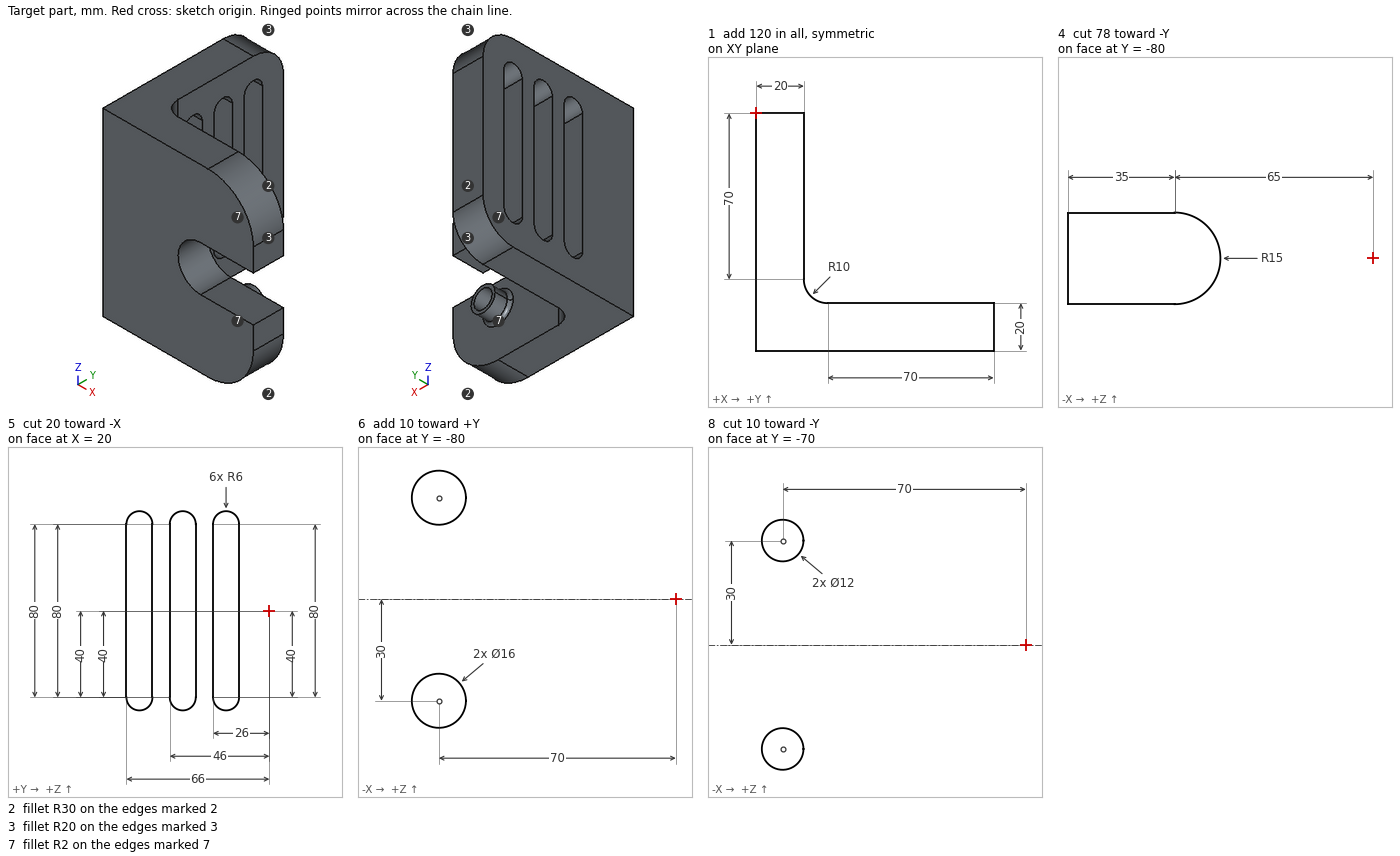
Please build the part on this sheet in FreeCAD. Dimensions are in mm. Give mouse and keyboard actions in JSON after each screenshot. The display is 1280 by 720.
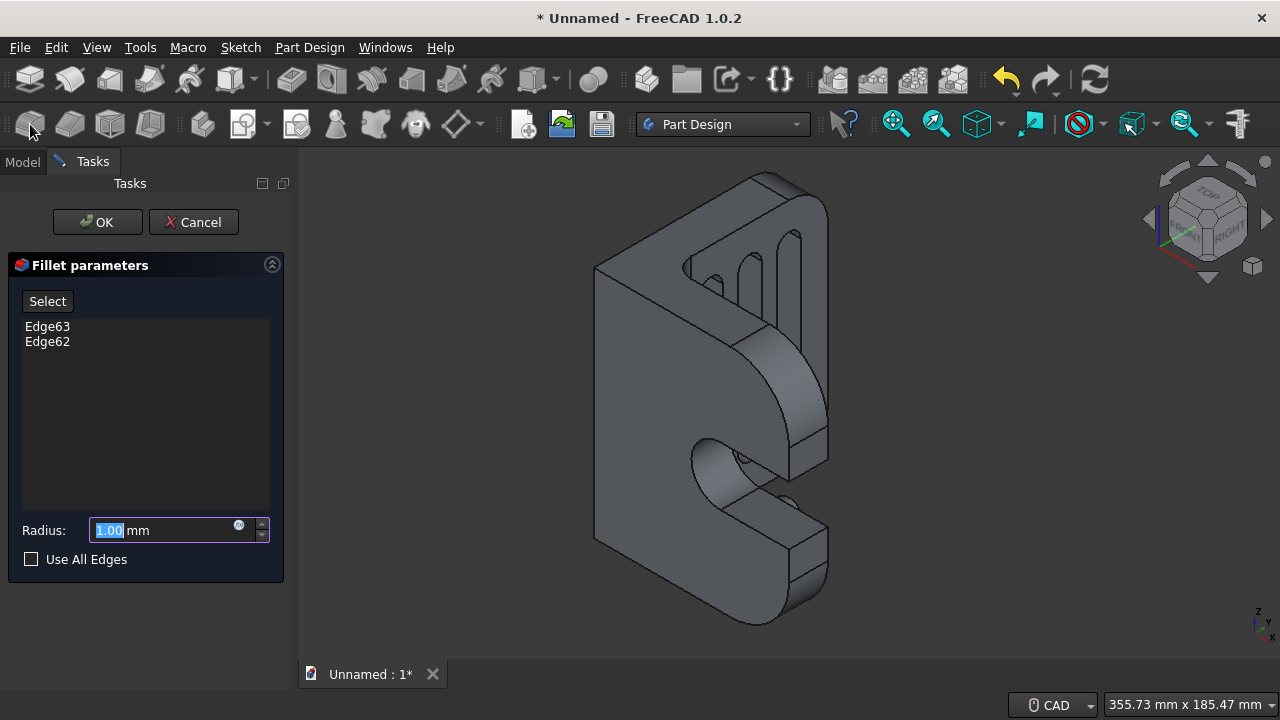
{"action": "type", "text": "2"}
{"action": "key", "text": "Tab"}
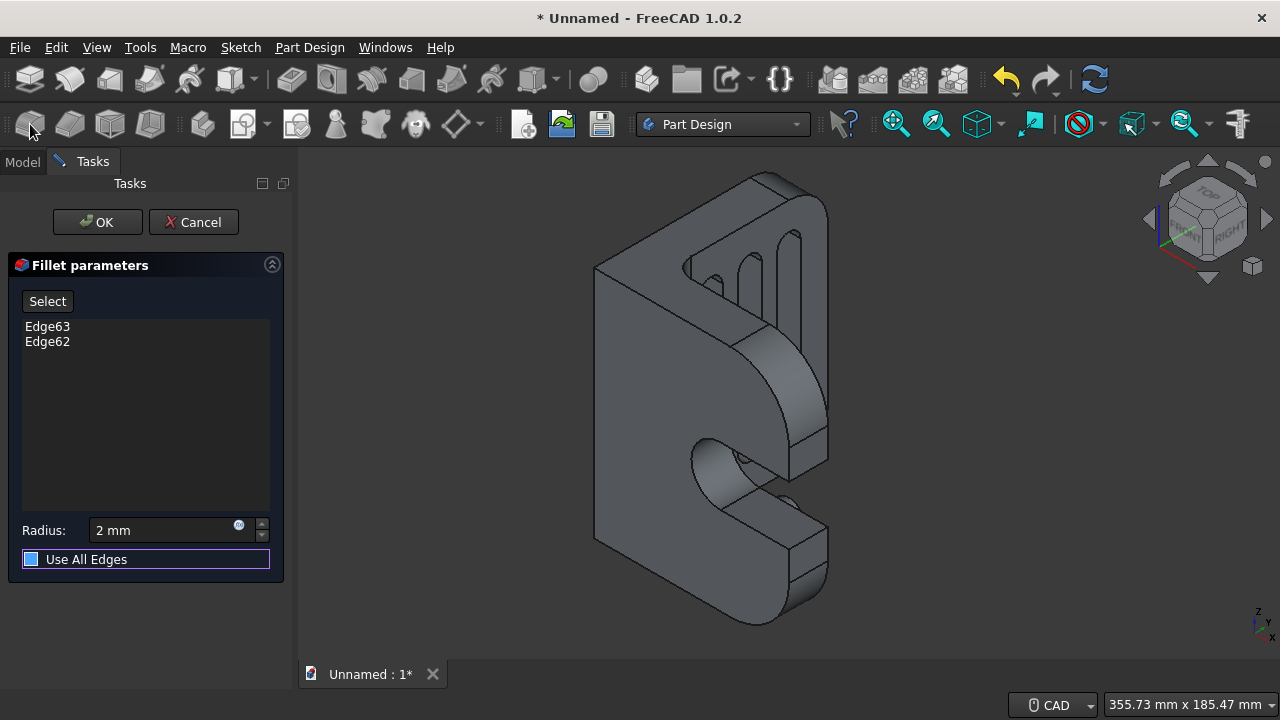
{"action": "left_click", "coordinate": [98, 222]}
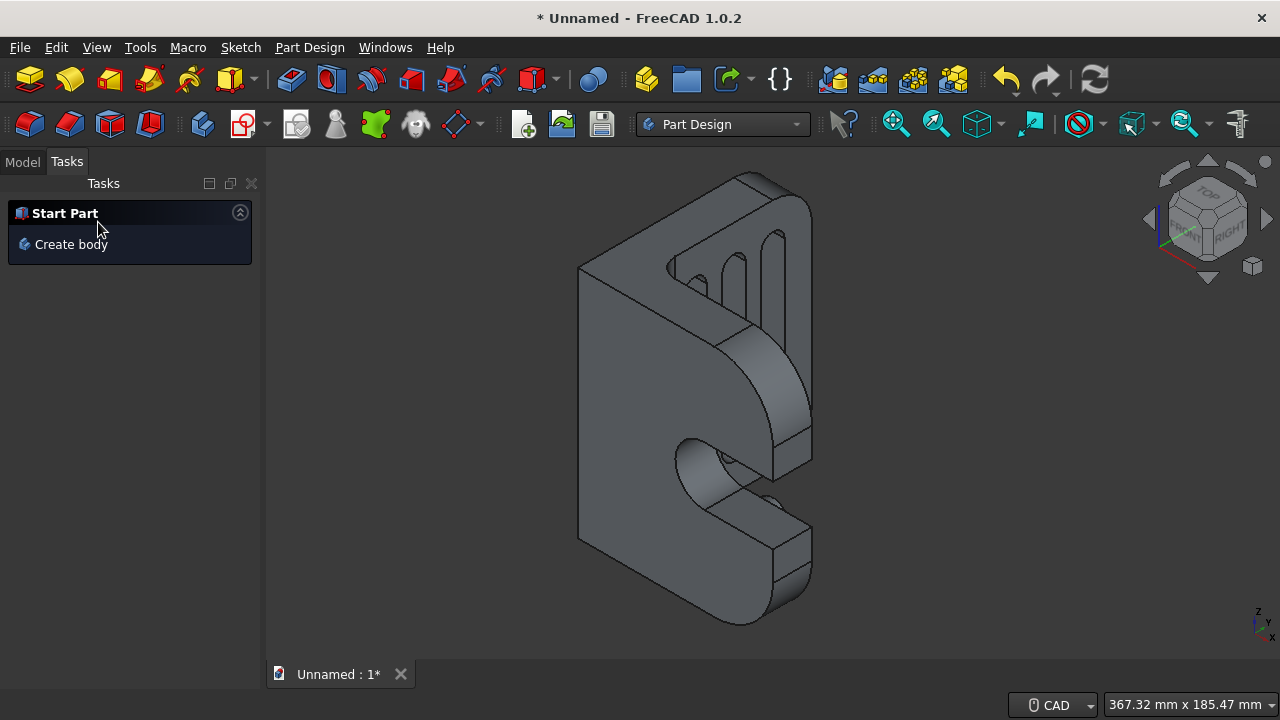
{"action": "key", "text": "4"}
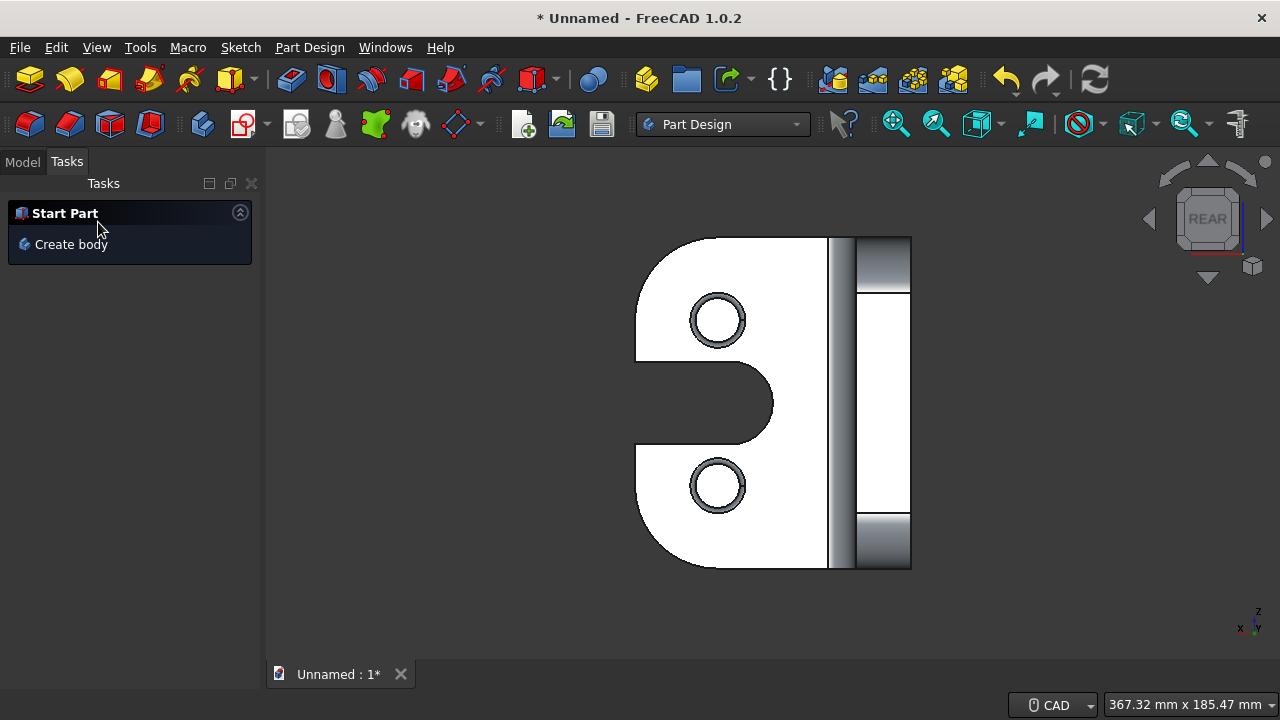
{"action": "left_click", "coordinate": [718, 319]}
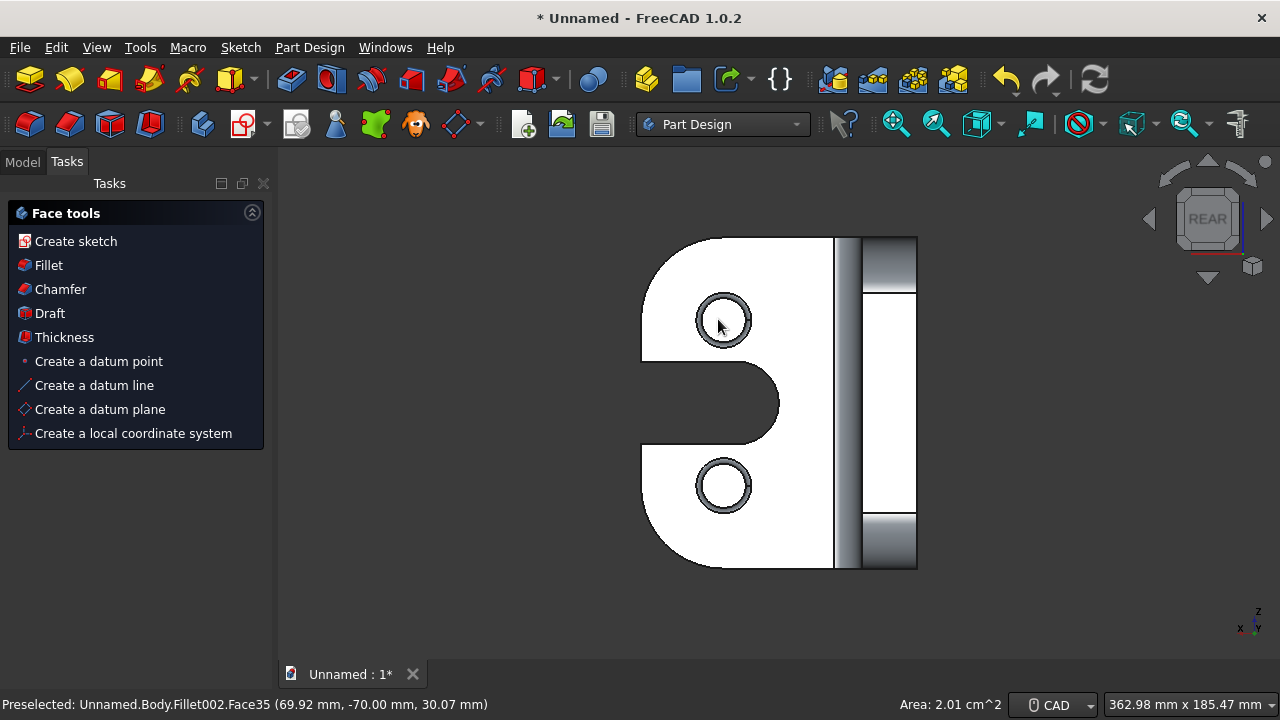
{"action": "left_click", "coordinate": [244, 124]}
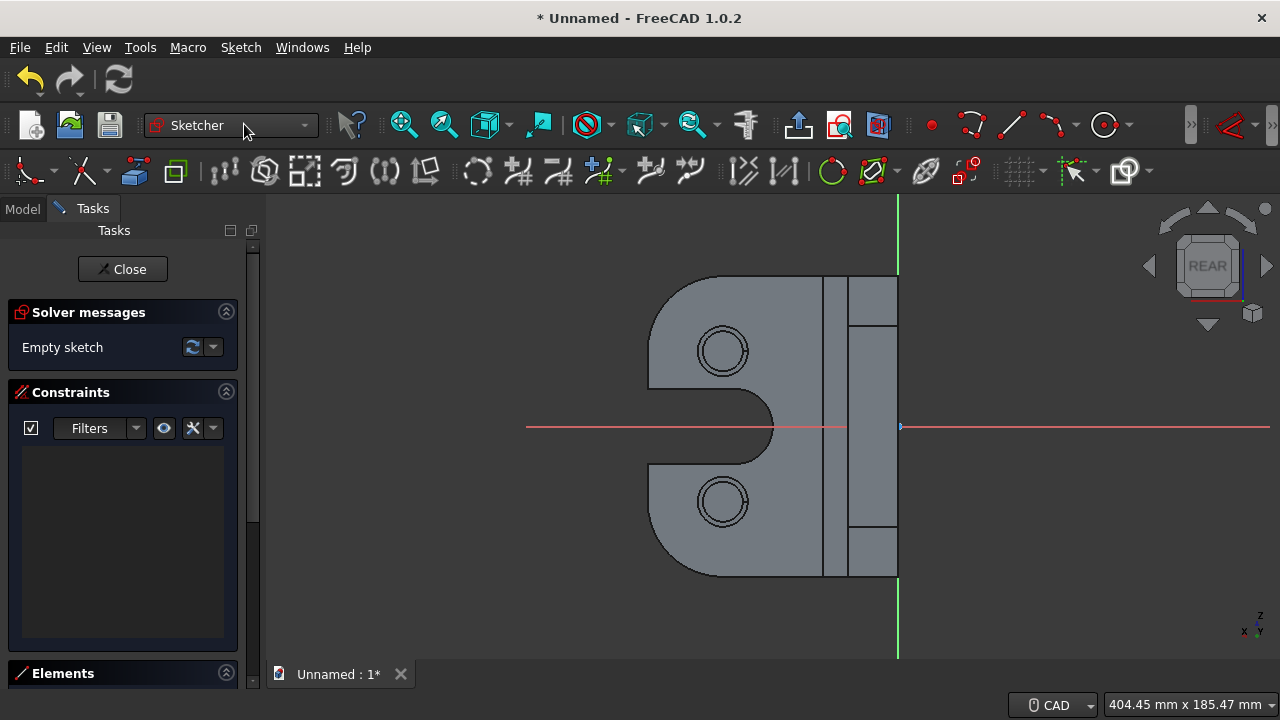
{"action": "key", "text": "q s"}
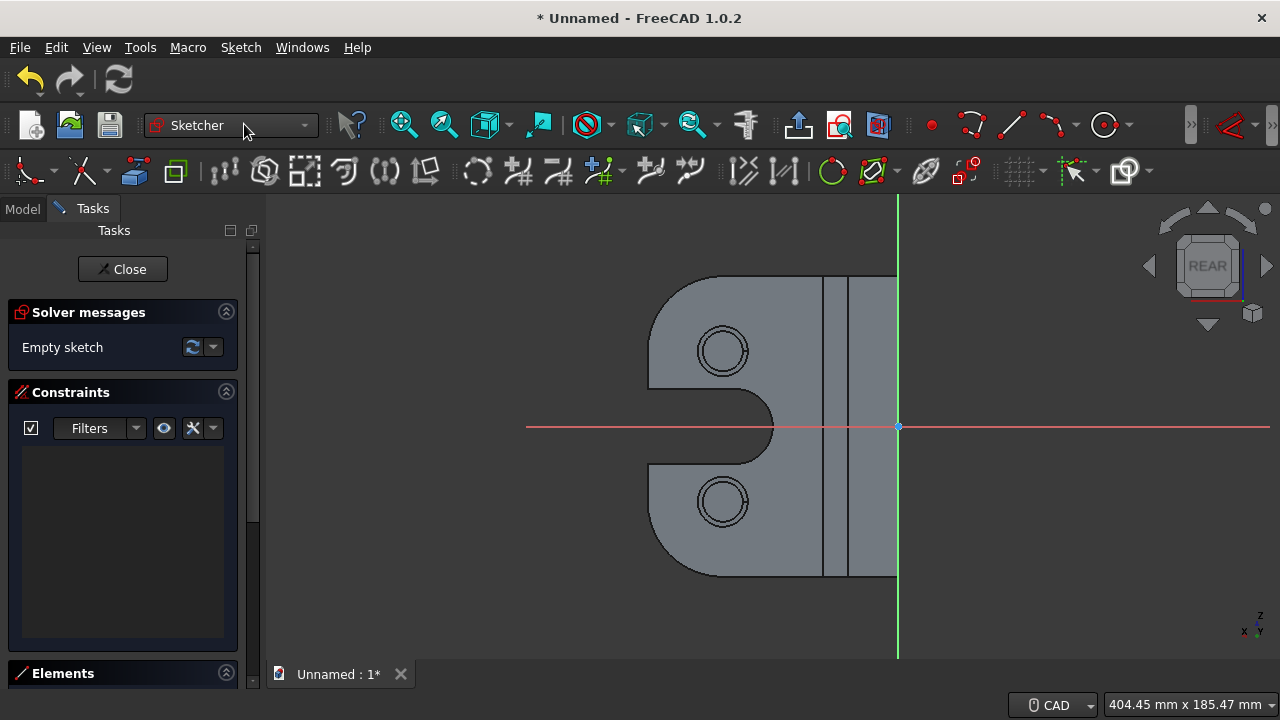
{"action": "scroll", "coordinate": [1004, 426], "scroll_direction": "up", "scroll_amount": 2}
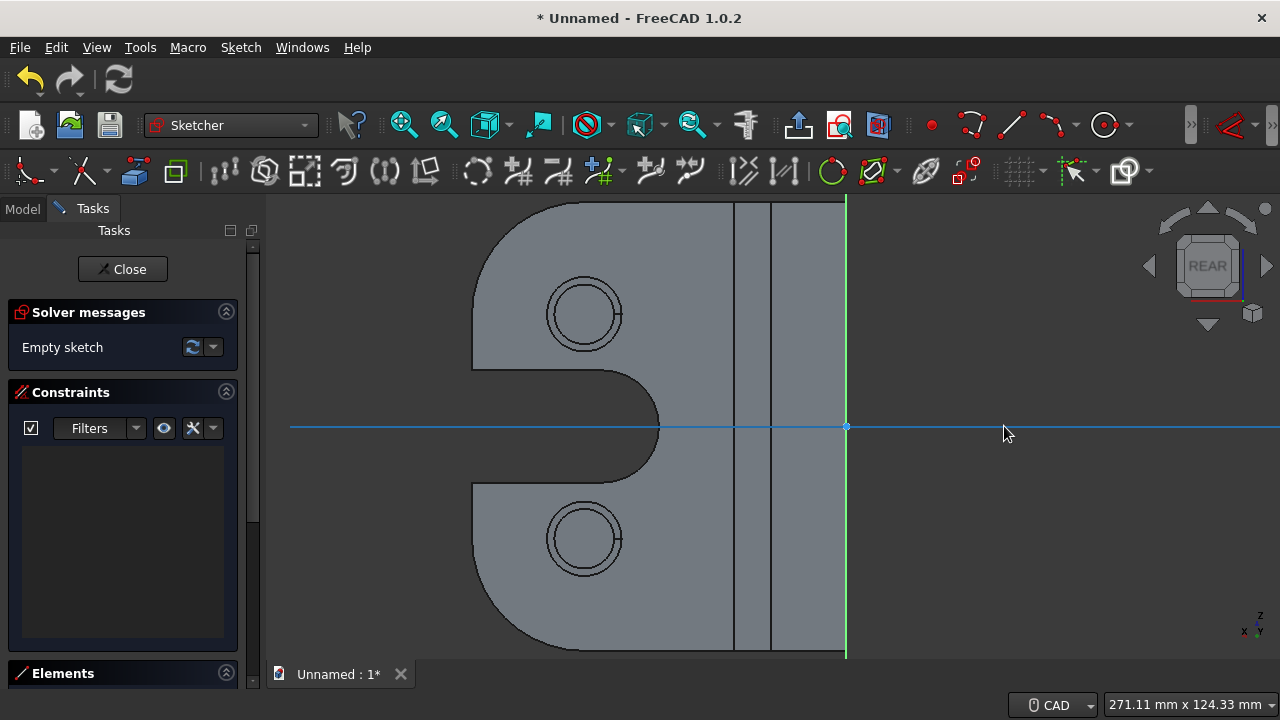
{"action": "key", "text": "g c"}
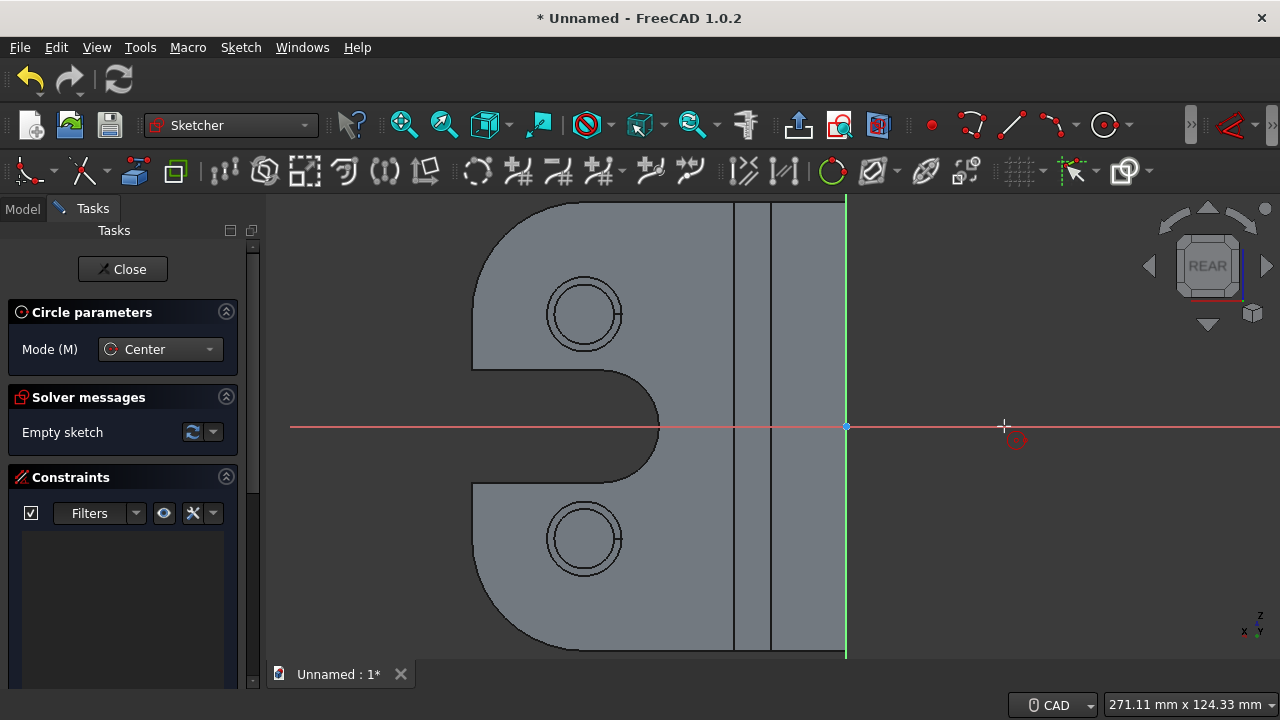
{"action": "left_click", "coordinate": [584, 314]}
{"action": "left_click", "coordinate": [600, 298]}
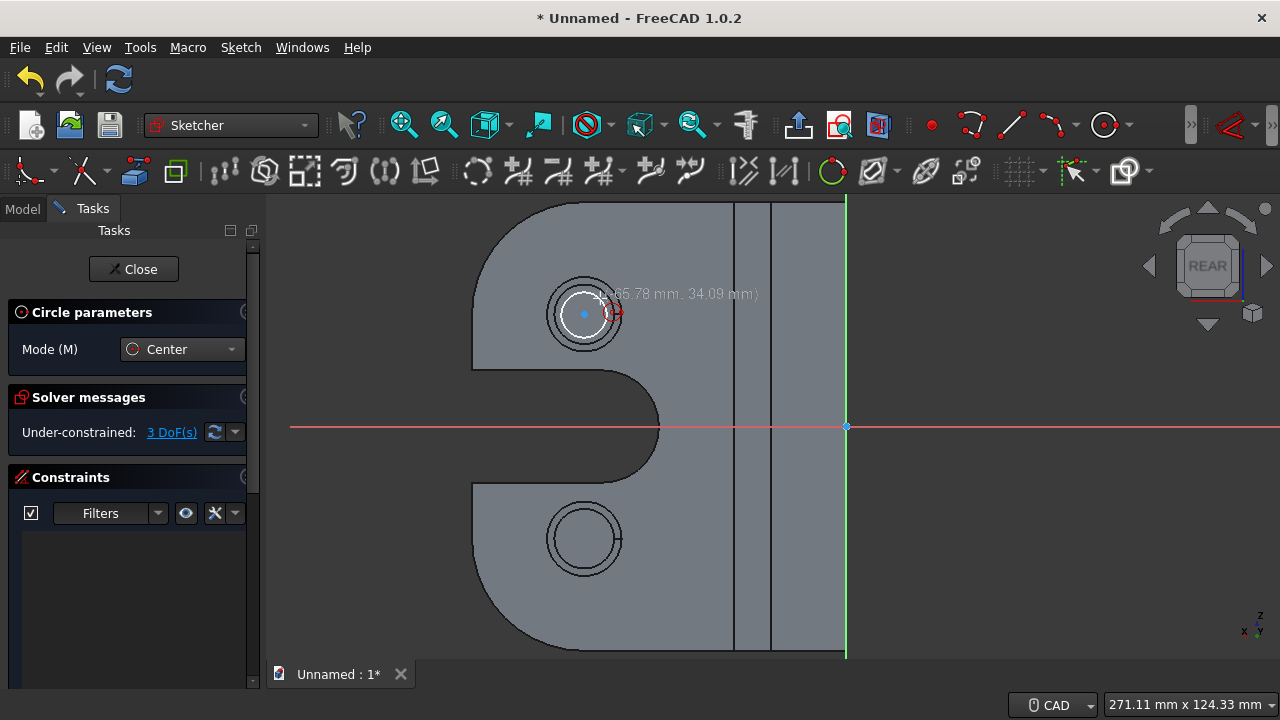
{"action": "left_click", "coordinate": [584, 539]}
{"action": "left_click", "coordinate": [600, 523]}
{"action": "key", "text": "Escape"}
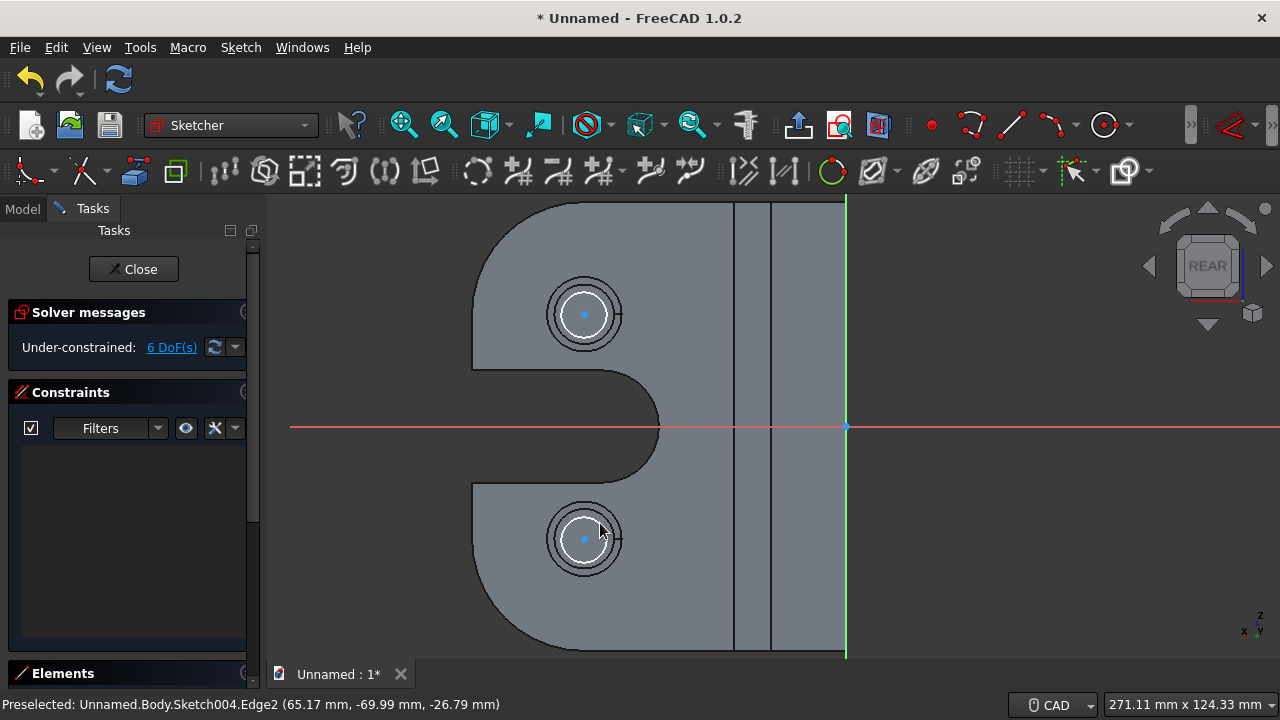
{"action": "left_click", "coordinate": [600, 299]}